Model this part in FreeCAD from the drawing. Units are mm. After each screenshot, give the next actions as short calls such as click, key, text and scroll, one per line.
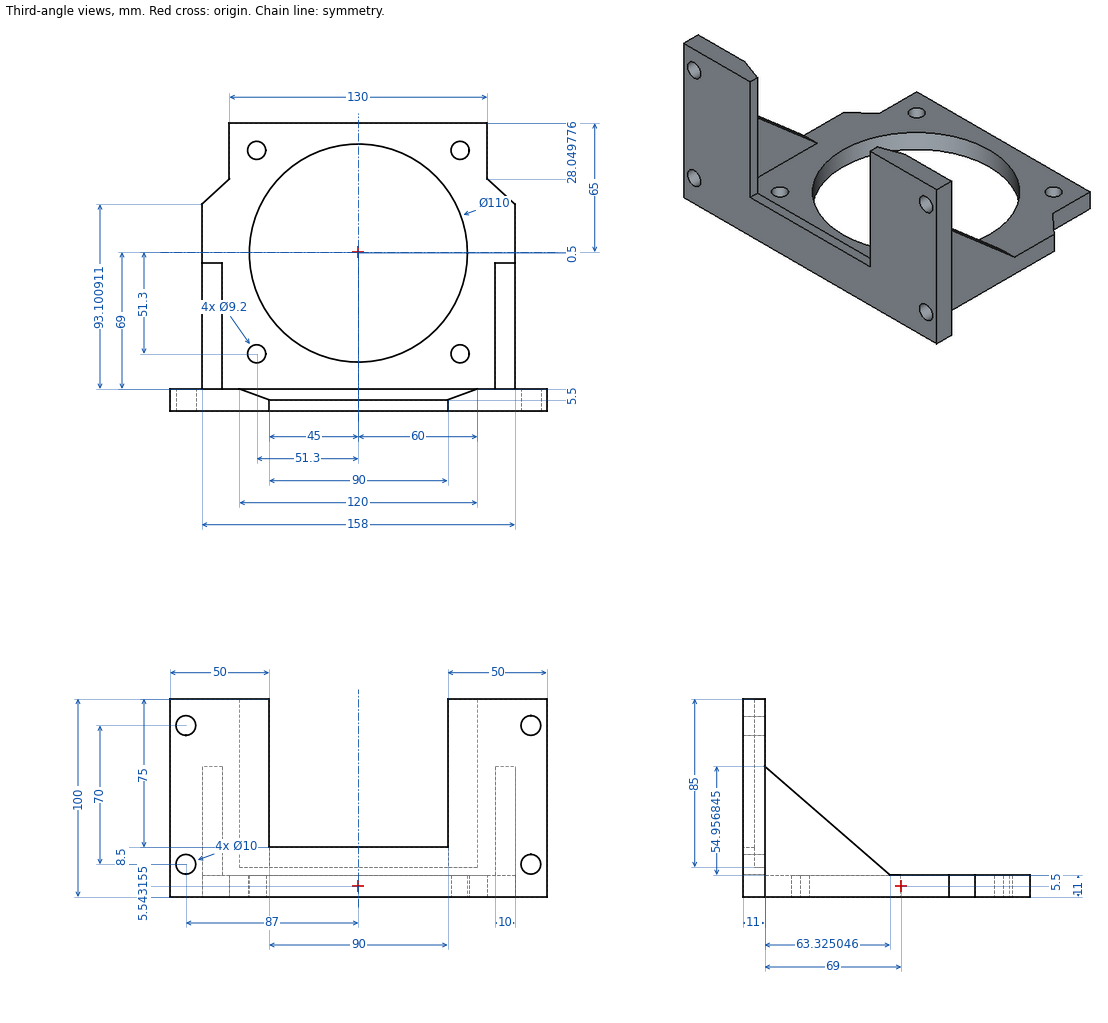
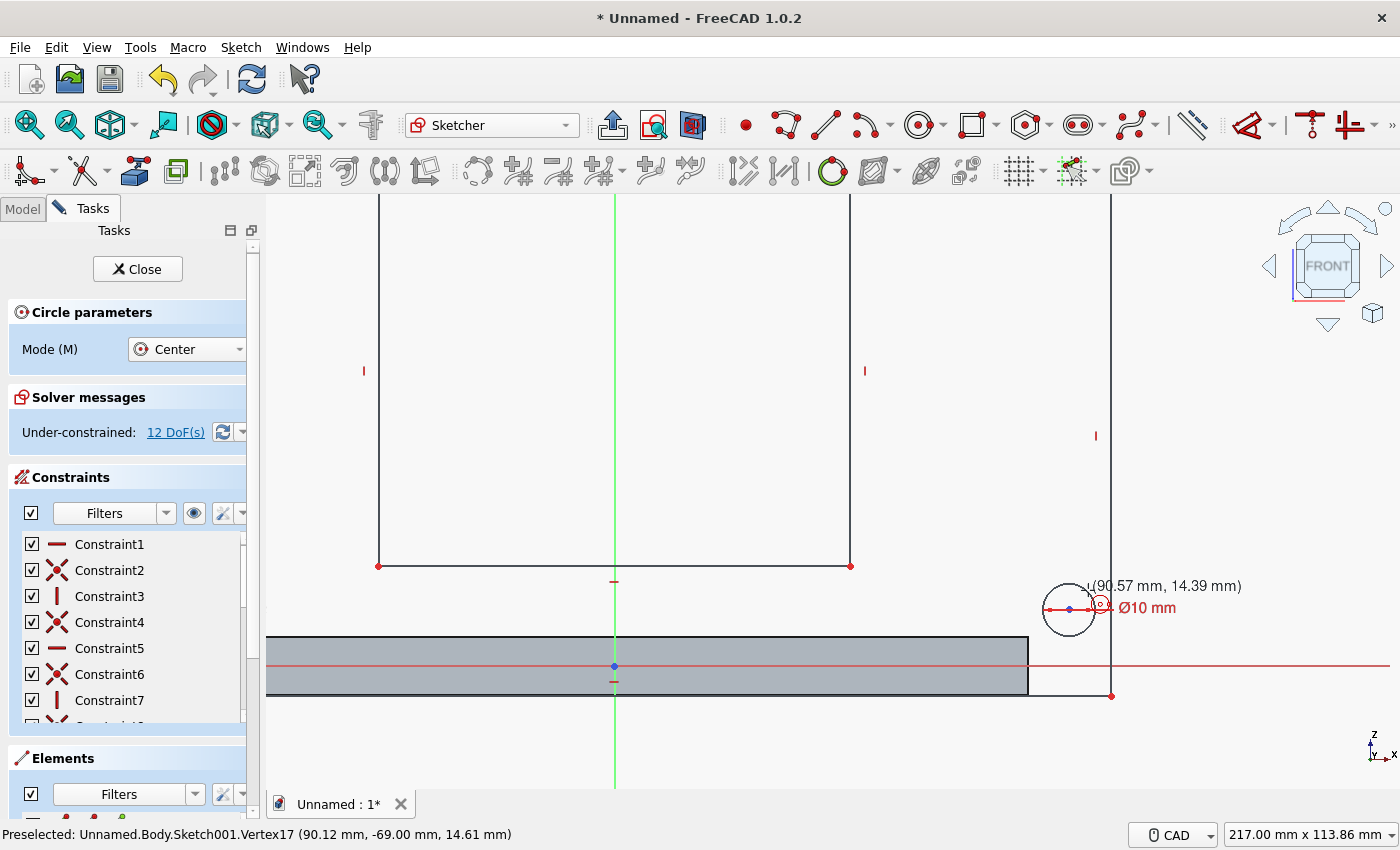
scroll(1069, 609, down, 2)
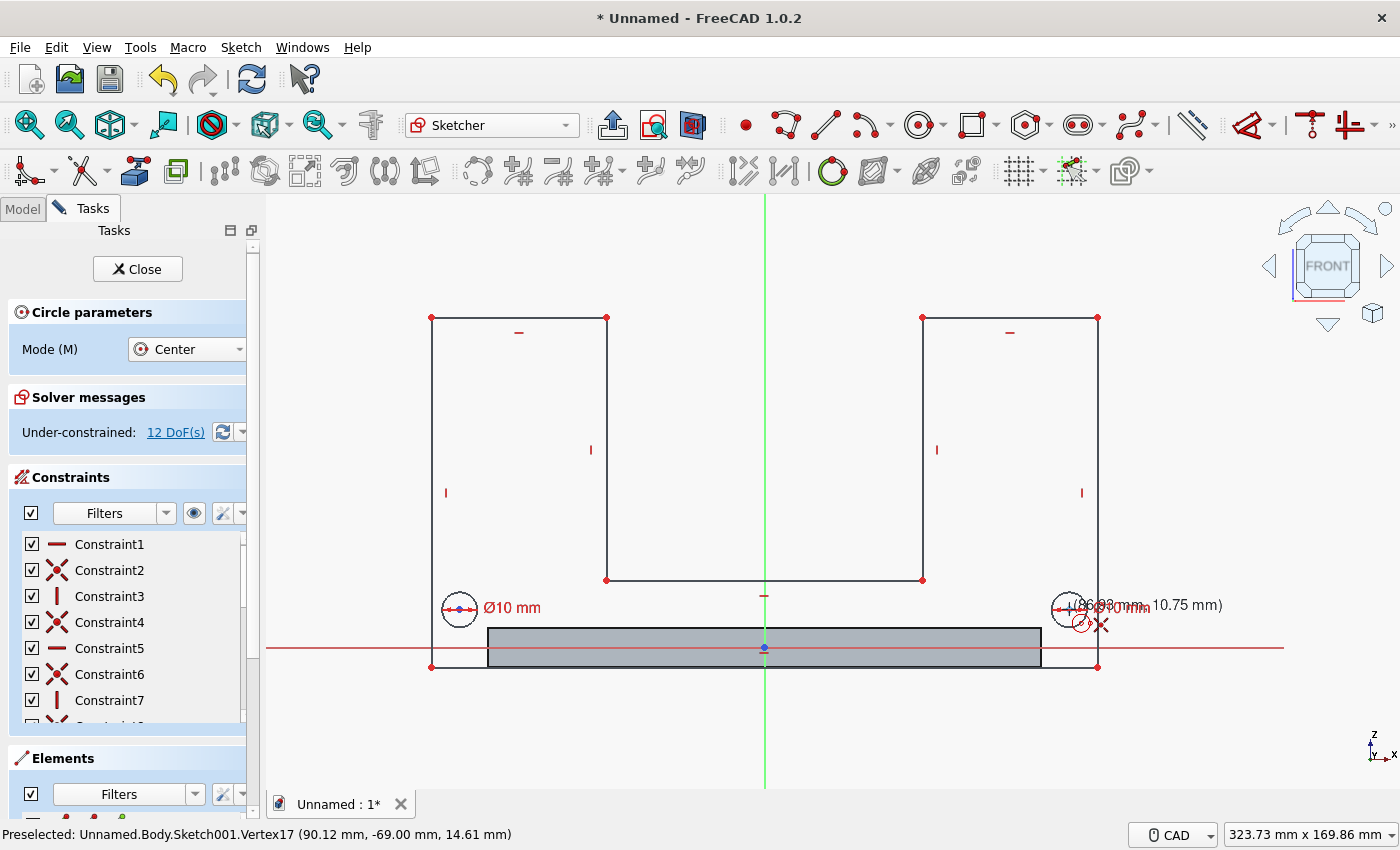
scroll(460, 364, up, 2)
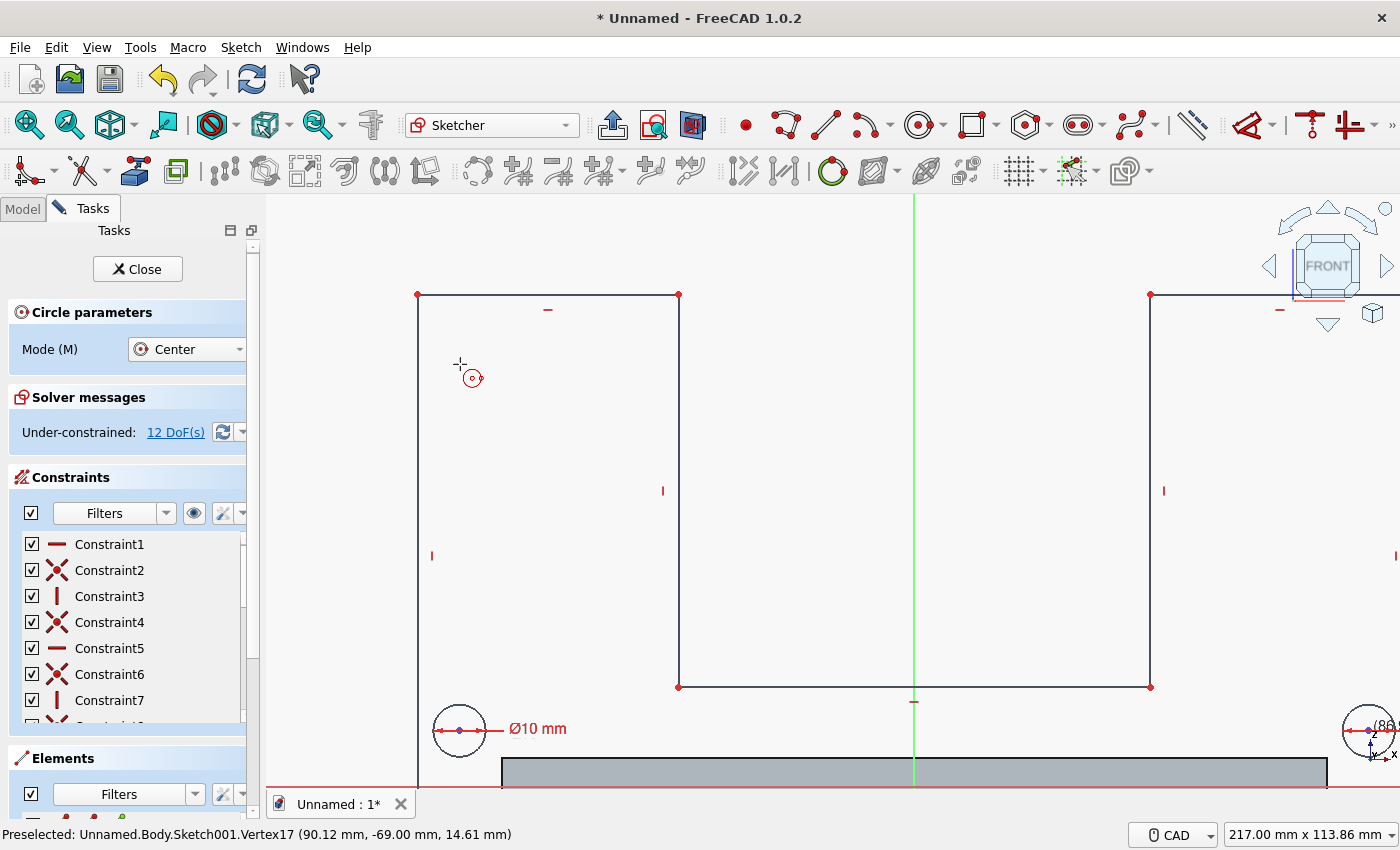
click(460, 364)
move(478, 345)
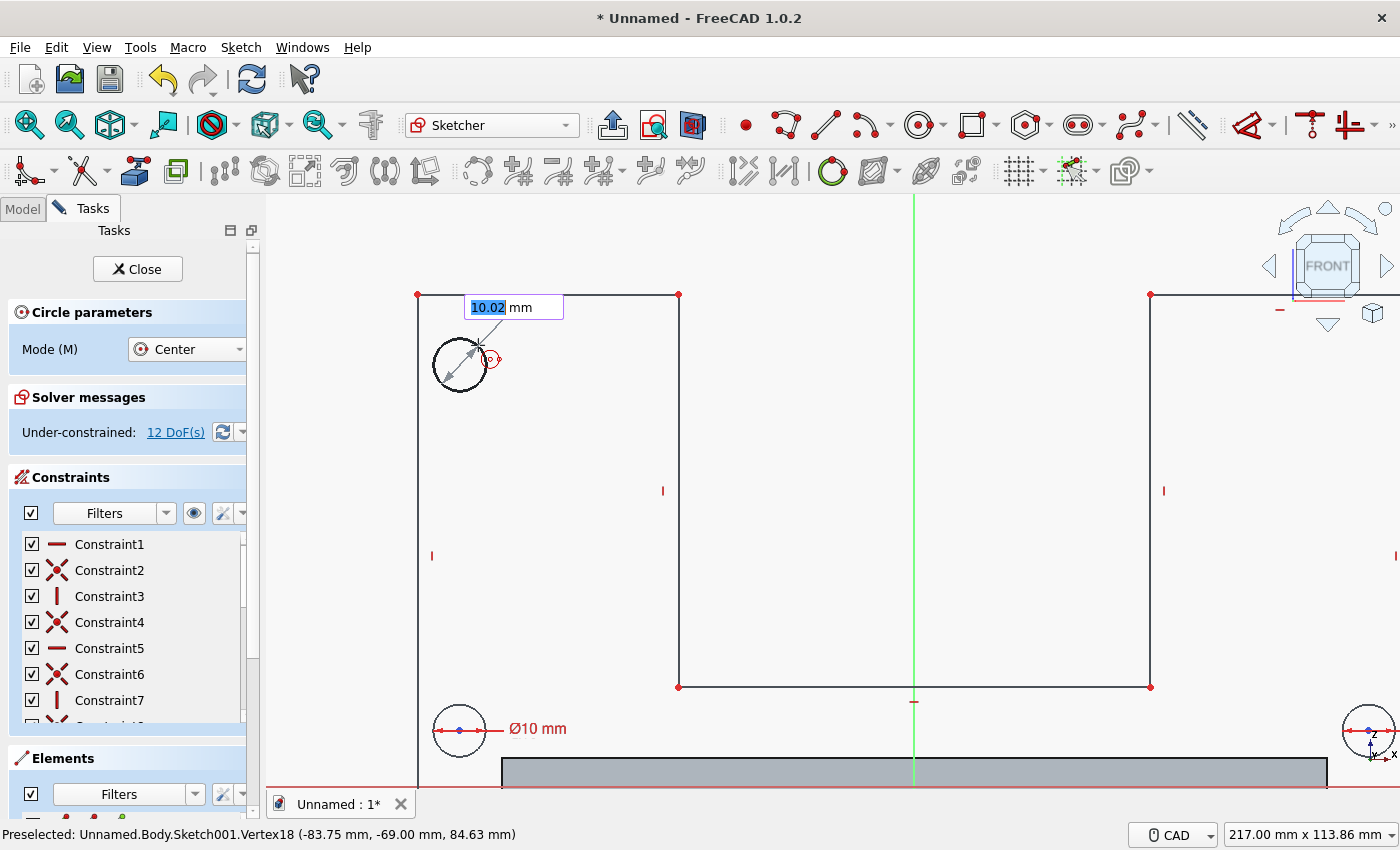
text(10)
key(Return)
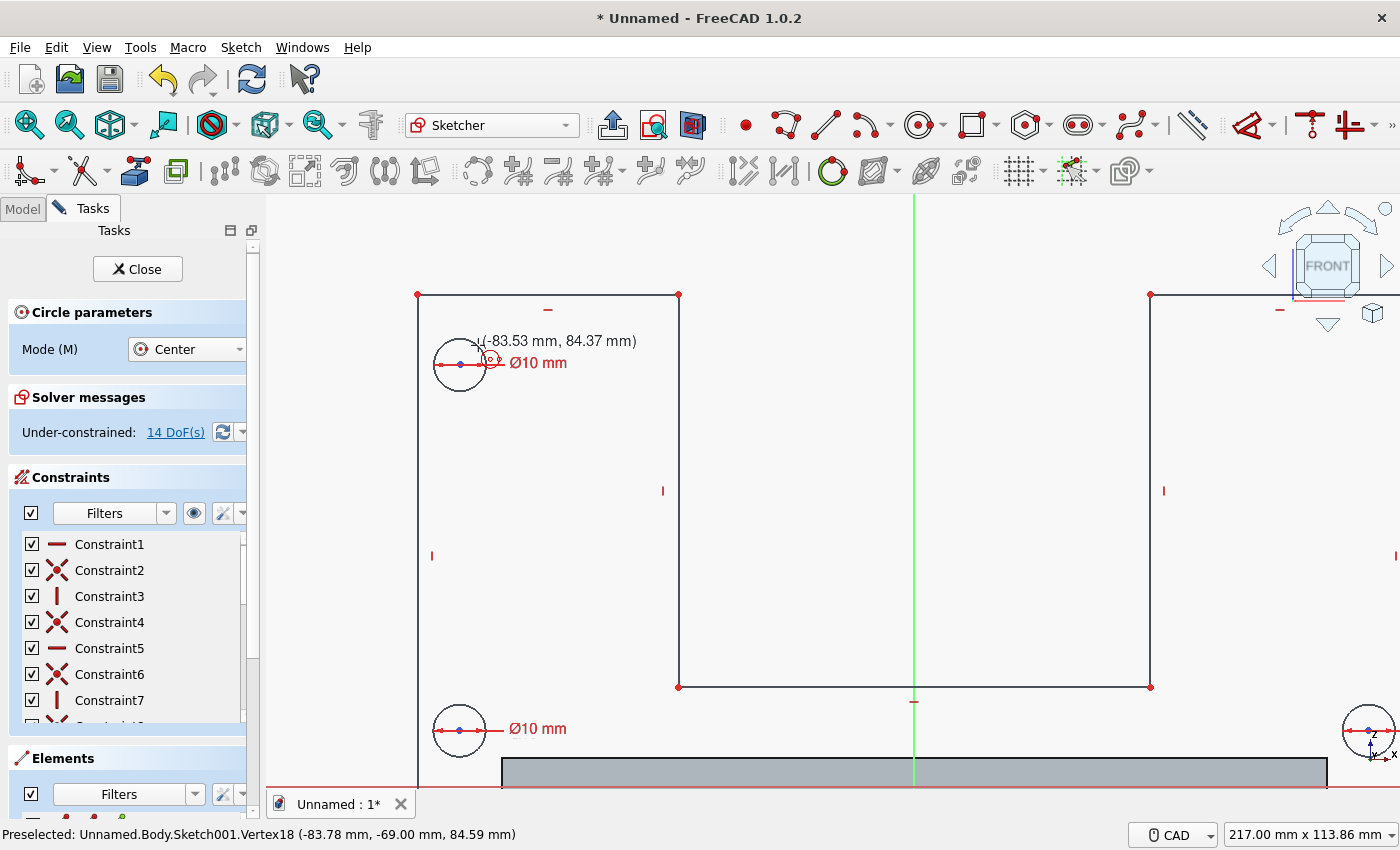
scroll(460, 363, down, 2)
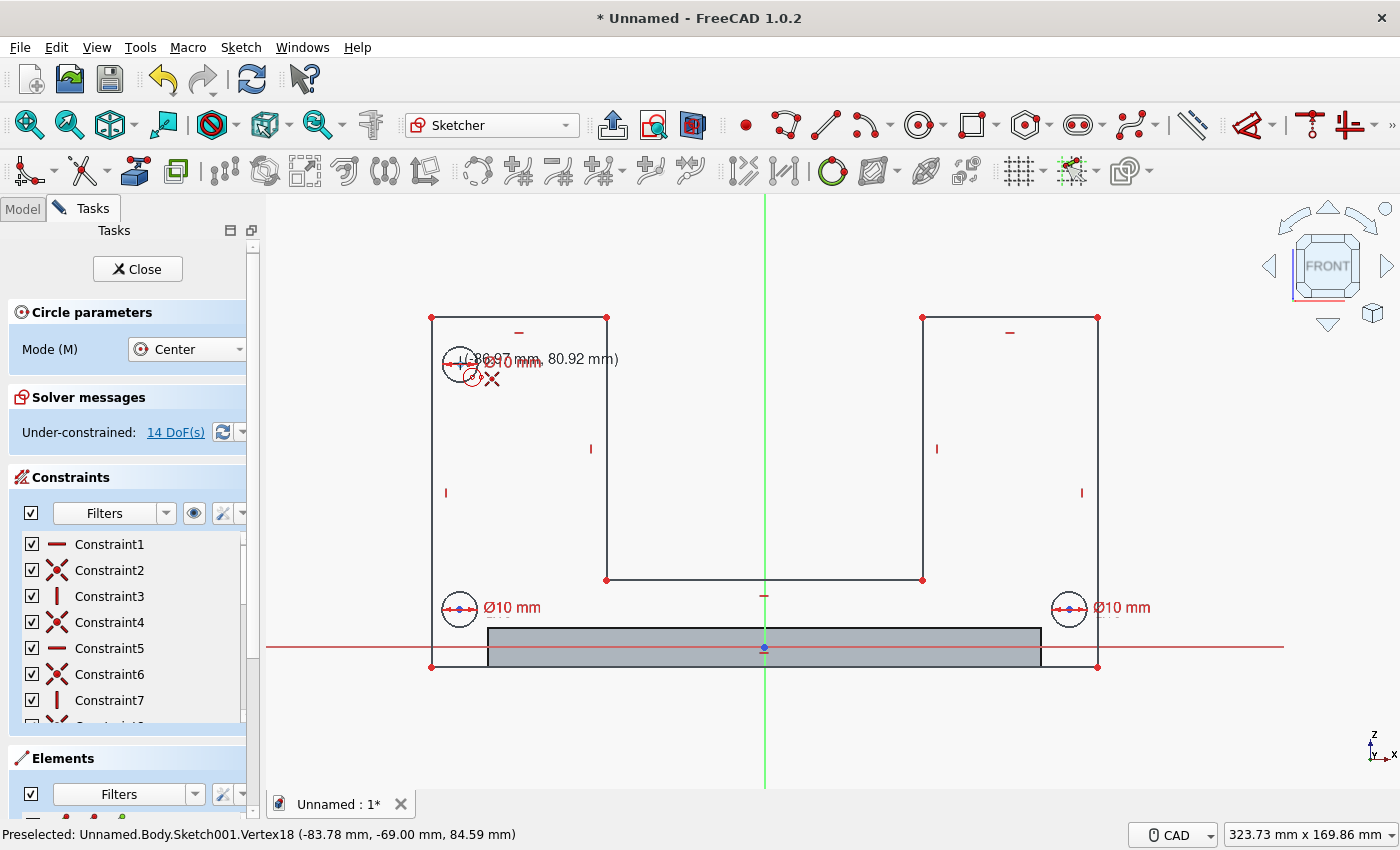
scroll(1069, 364, up, 2)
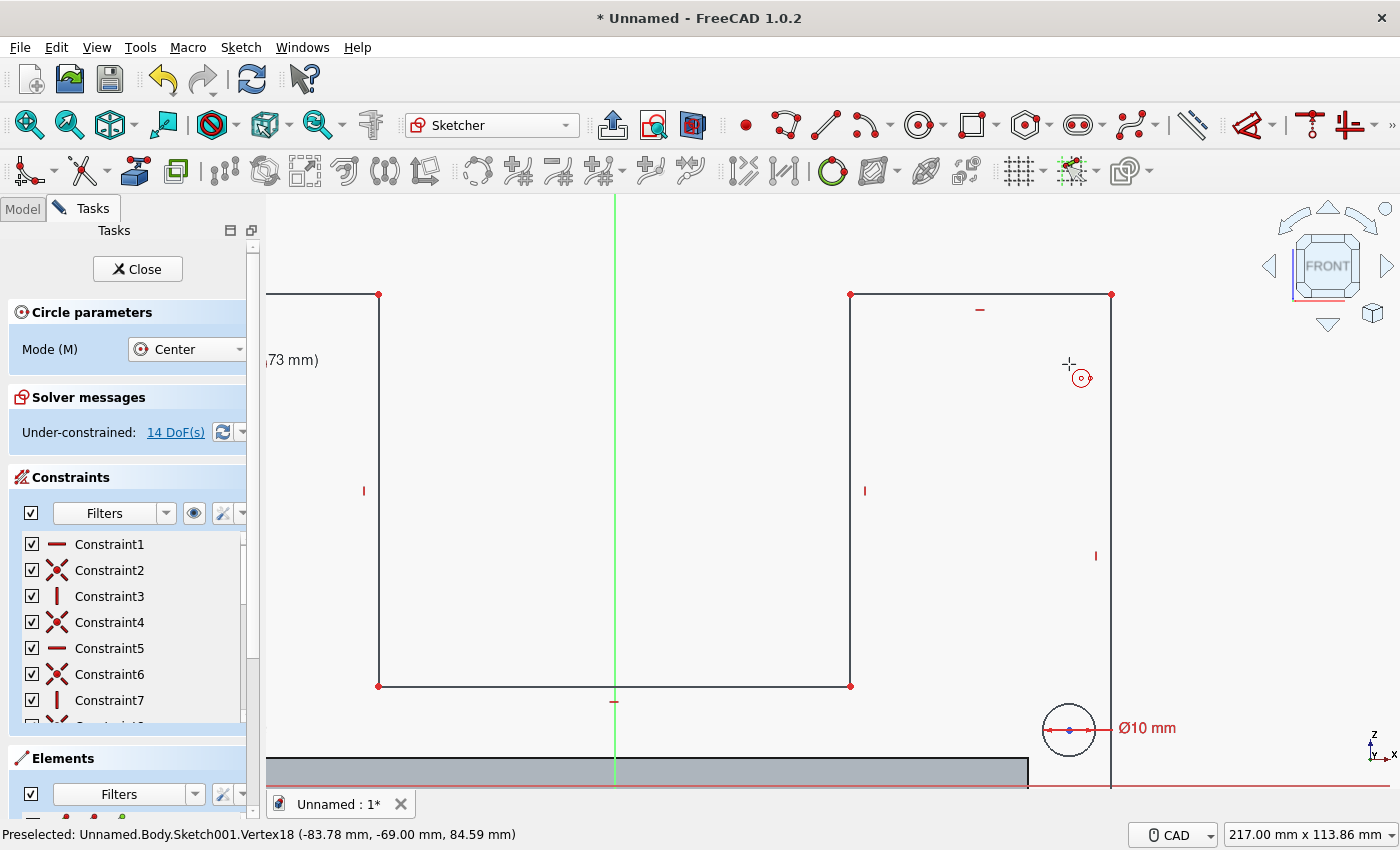
click(1069, 363)
move(1088, 345)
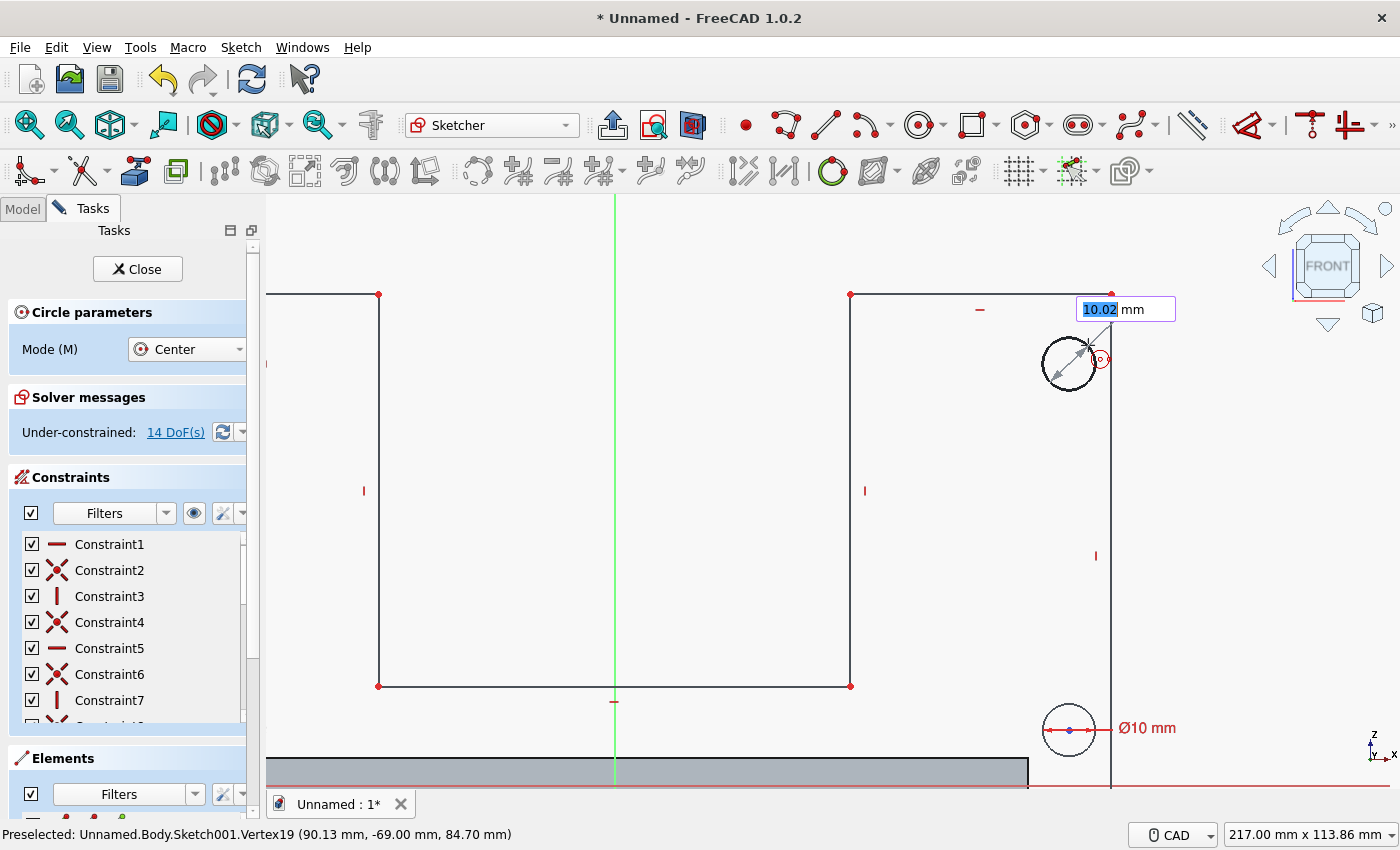
text(10)
key(Return)
key(Escape)